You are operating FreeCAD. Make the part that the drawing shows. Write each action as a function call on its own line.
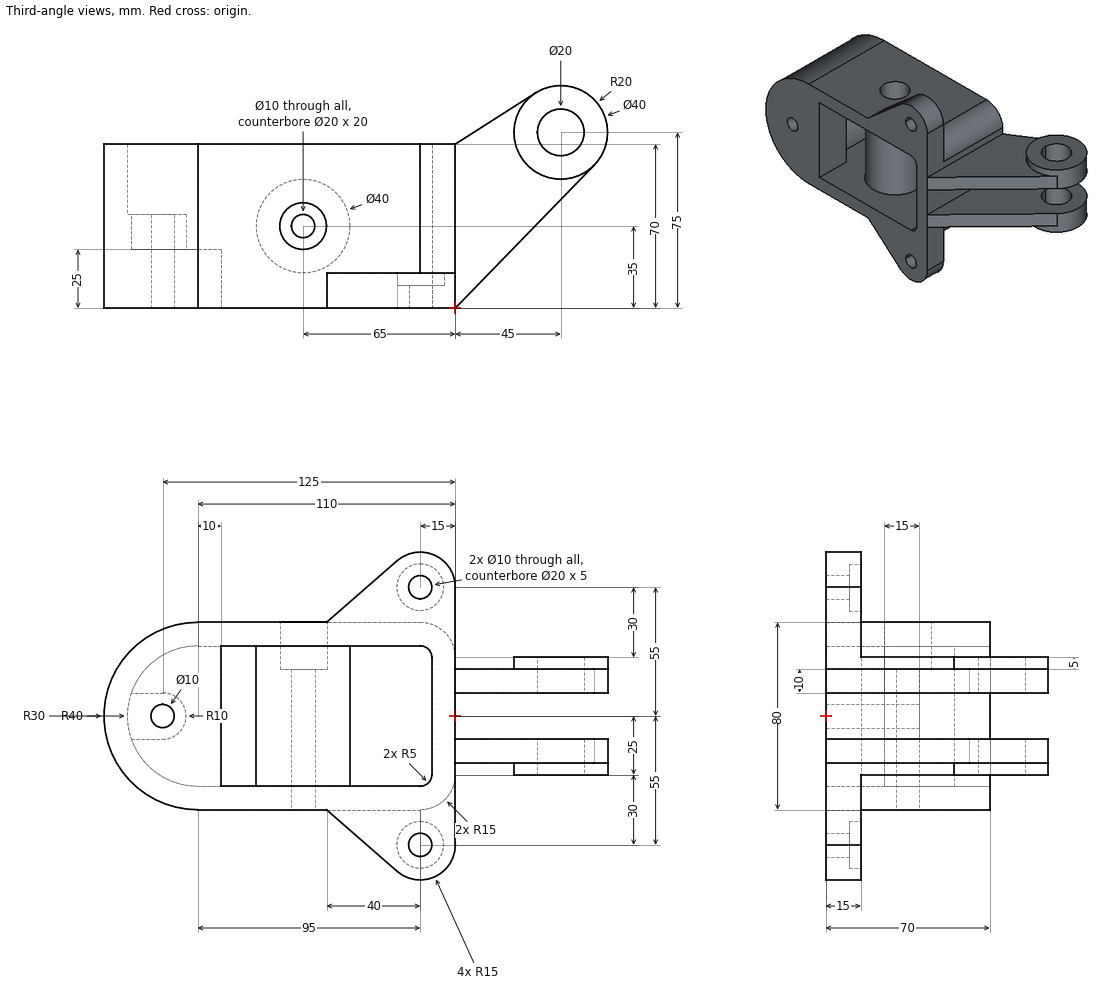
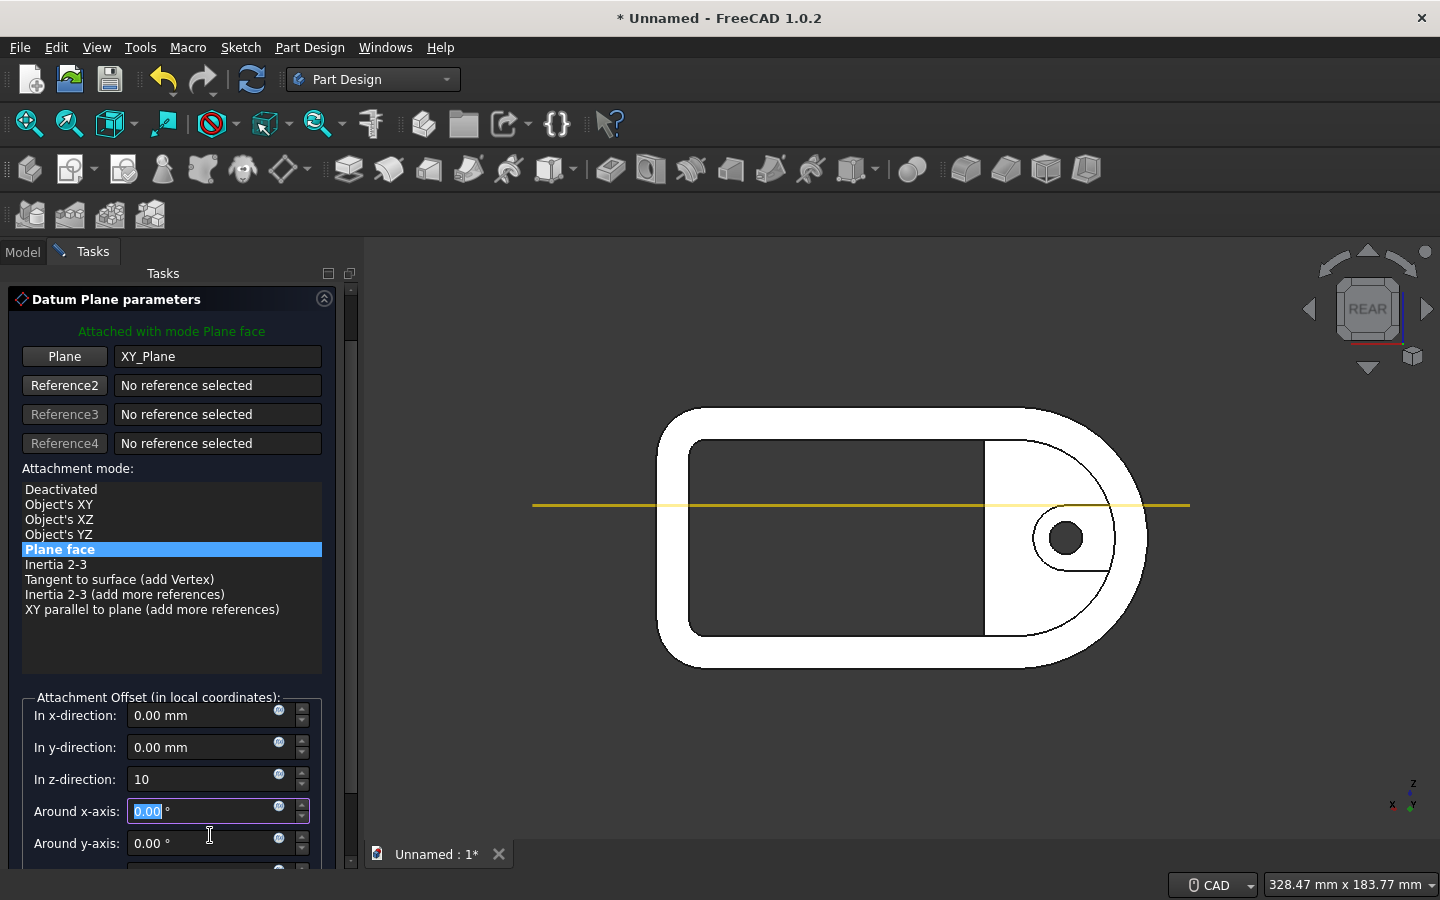
scroll(351, 576, up, 2)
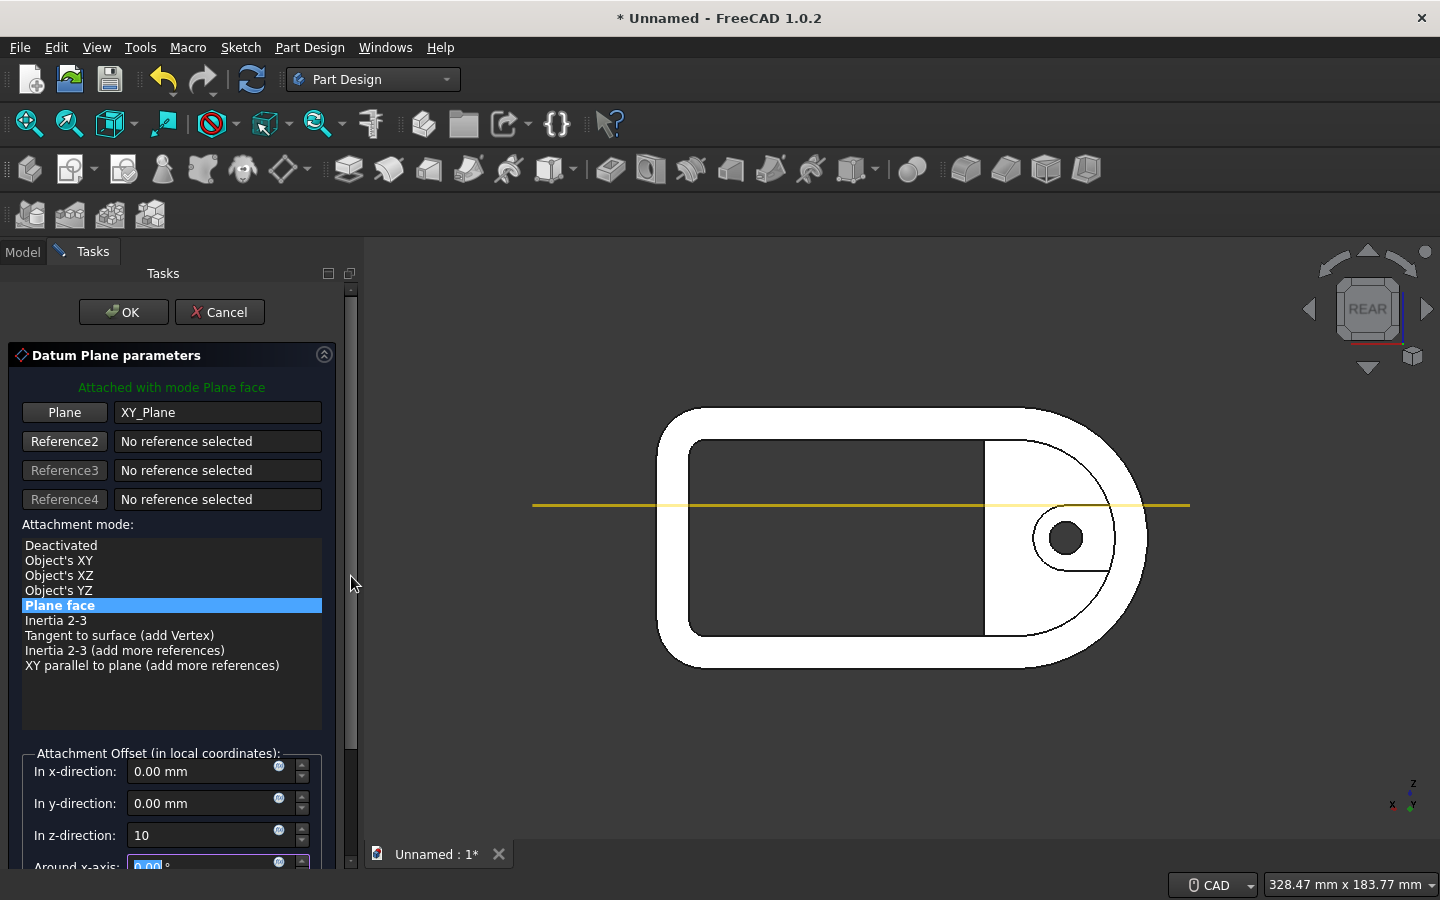
click(124, 312)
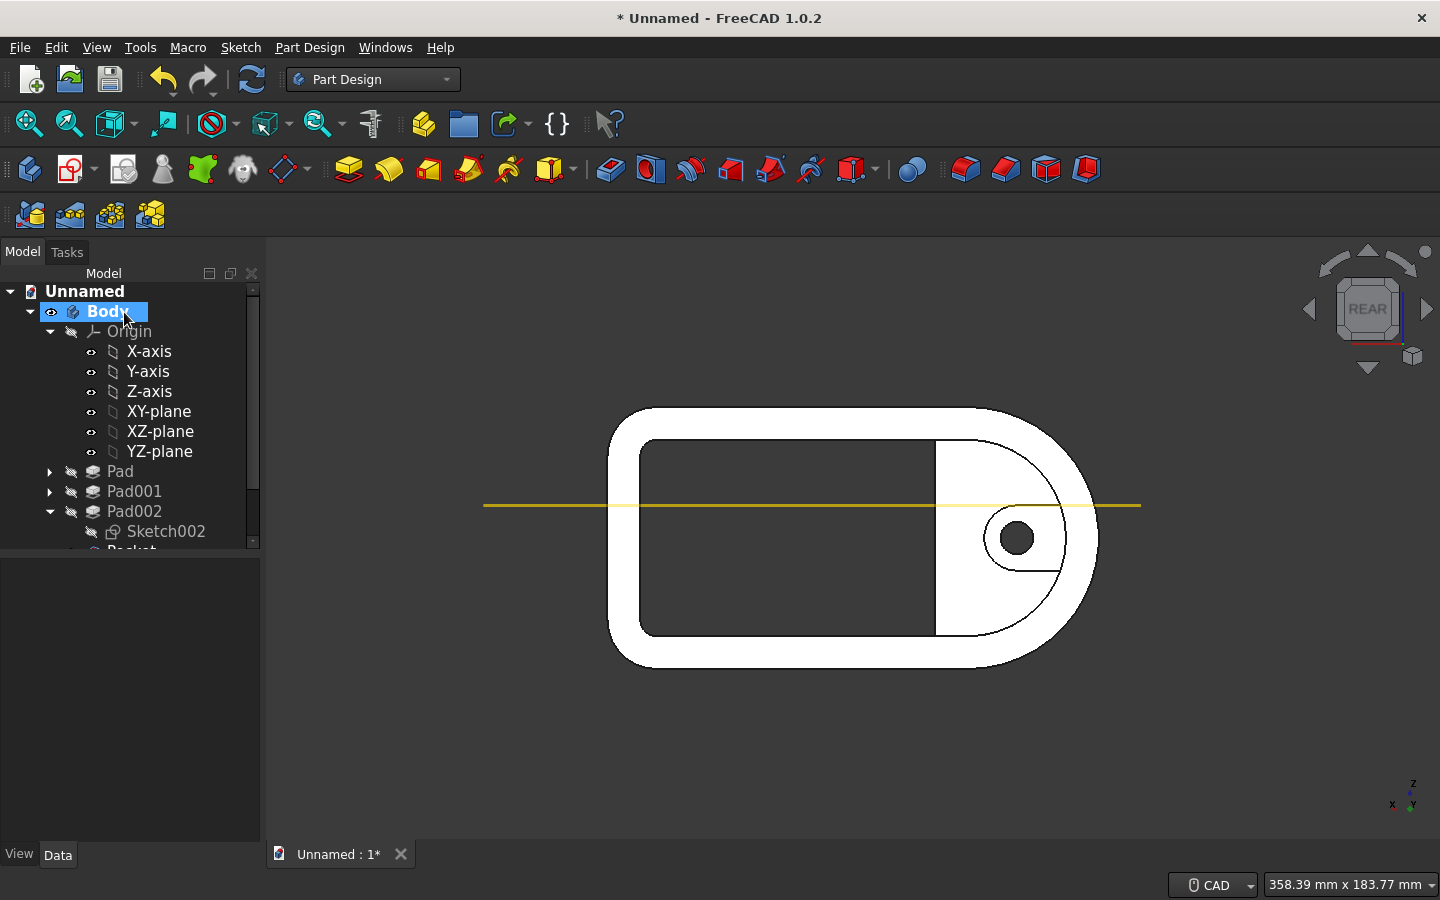
scroll(100, 407, down, 3)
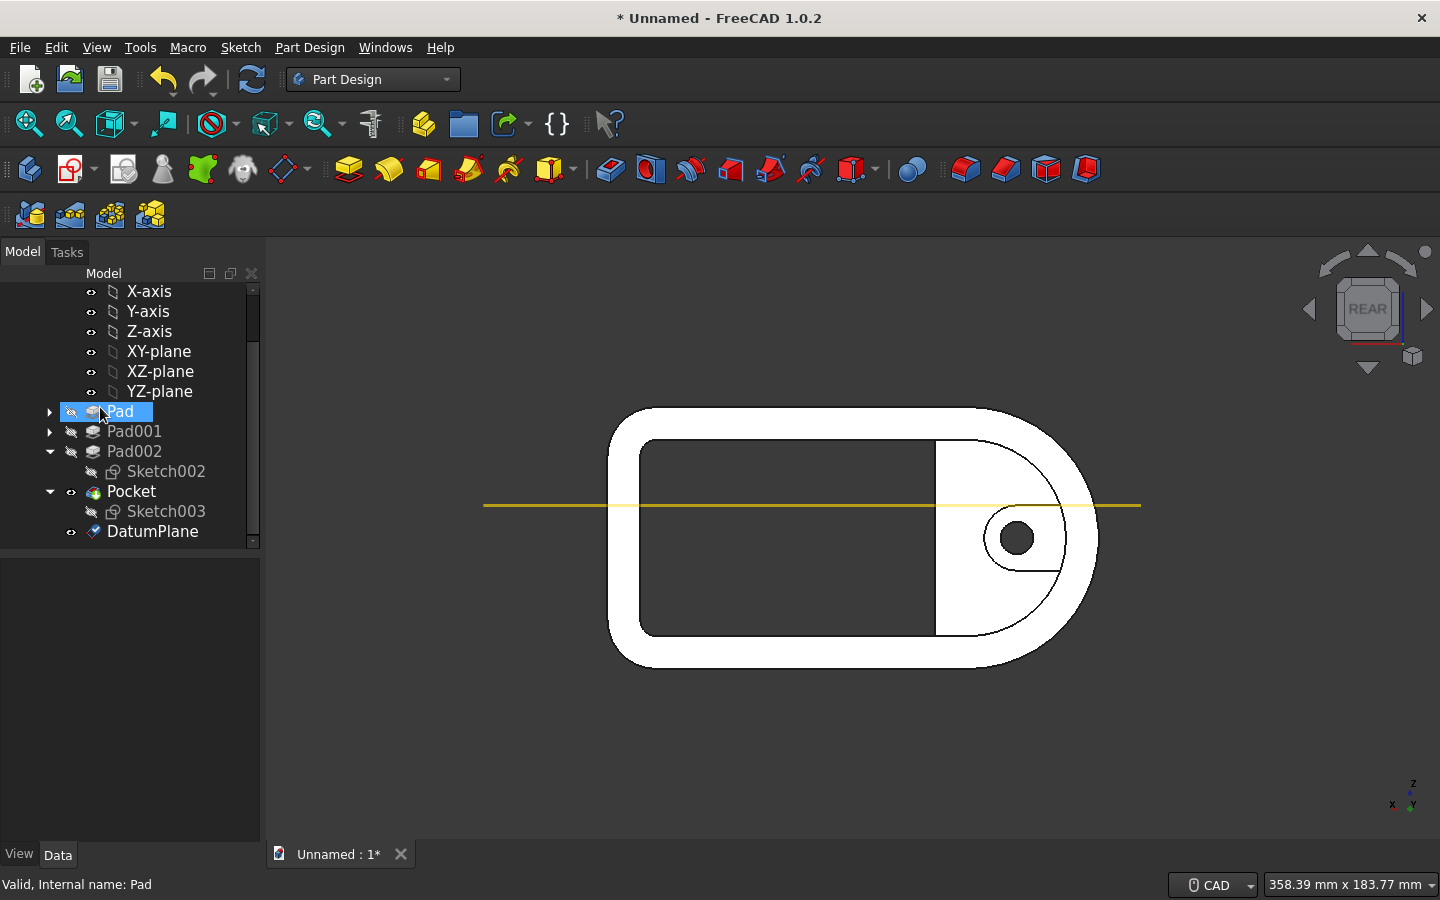
click(116, 532)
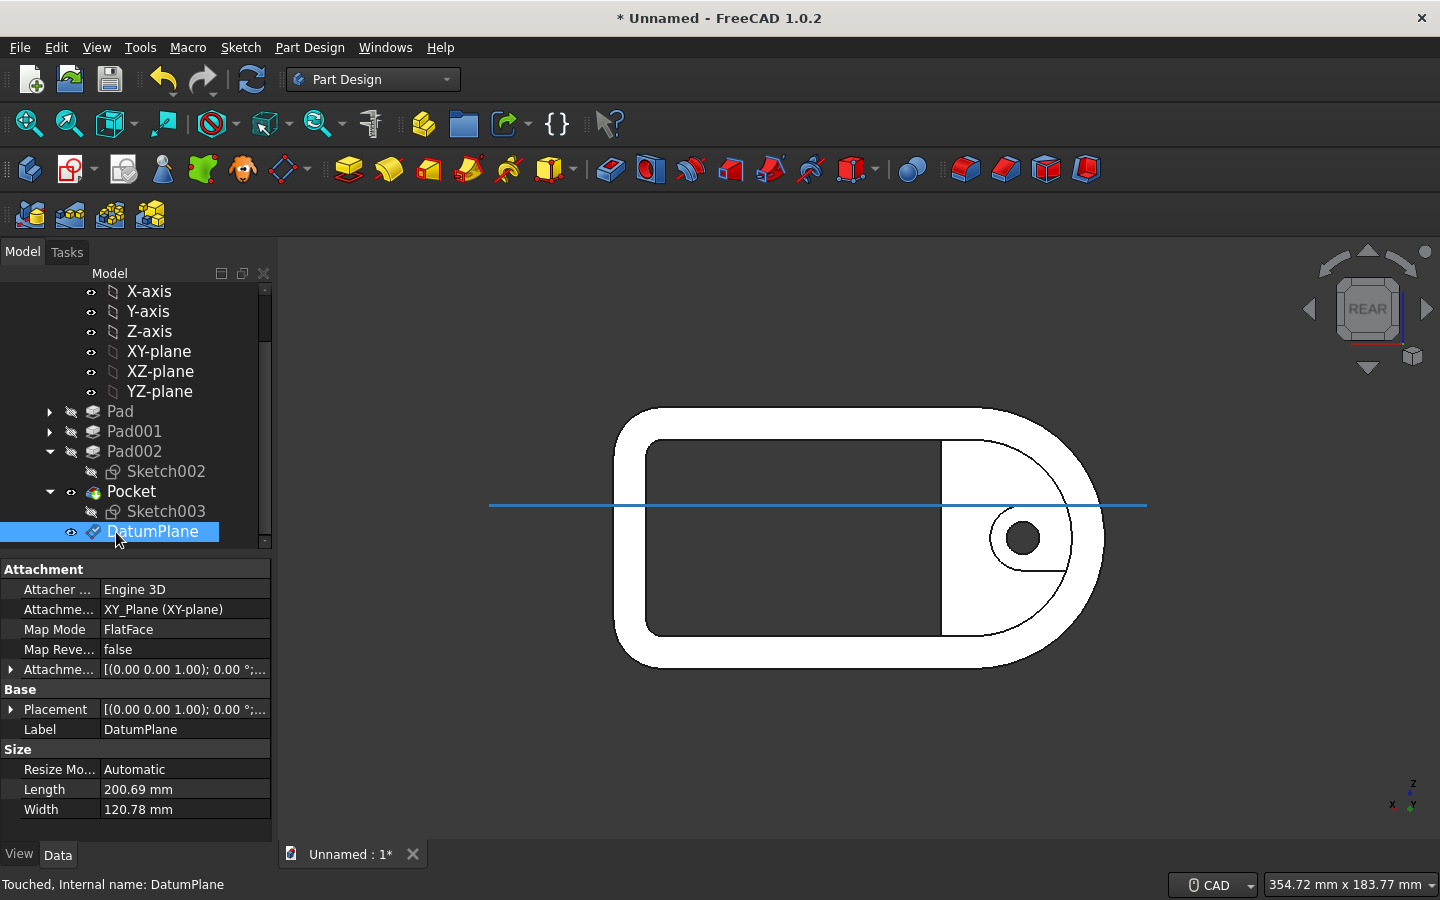
click(70, 170)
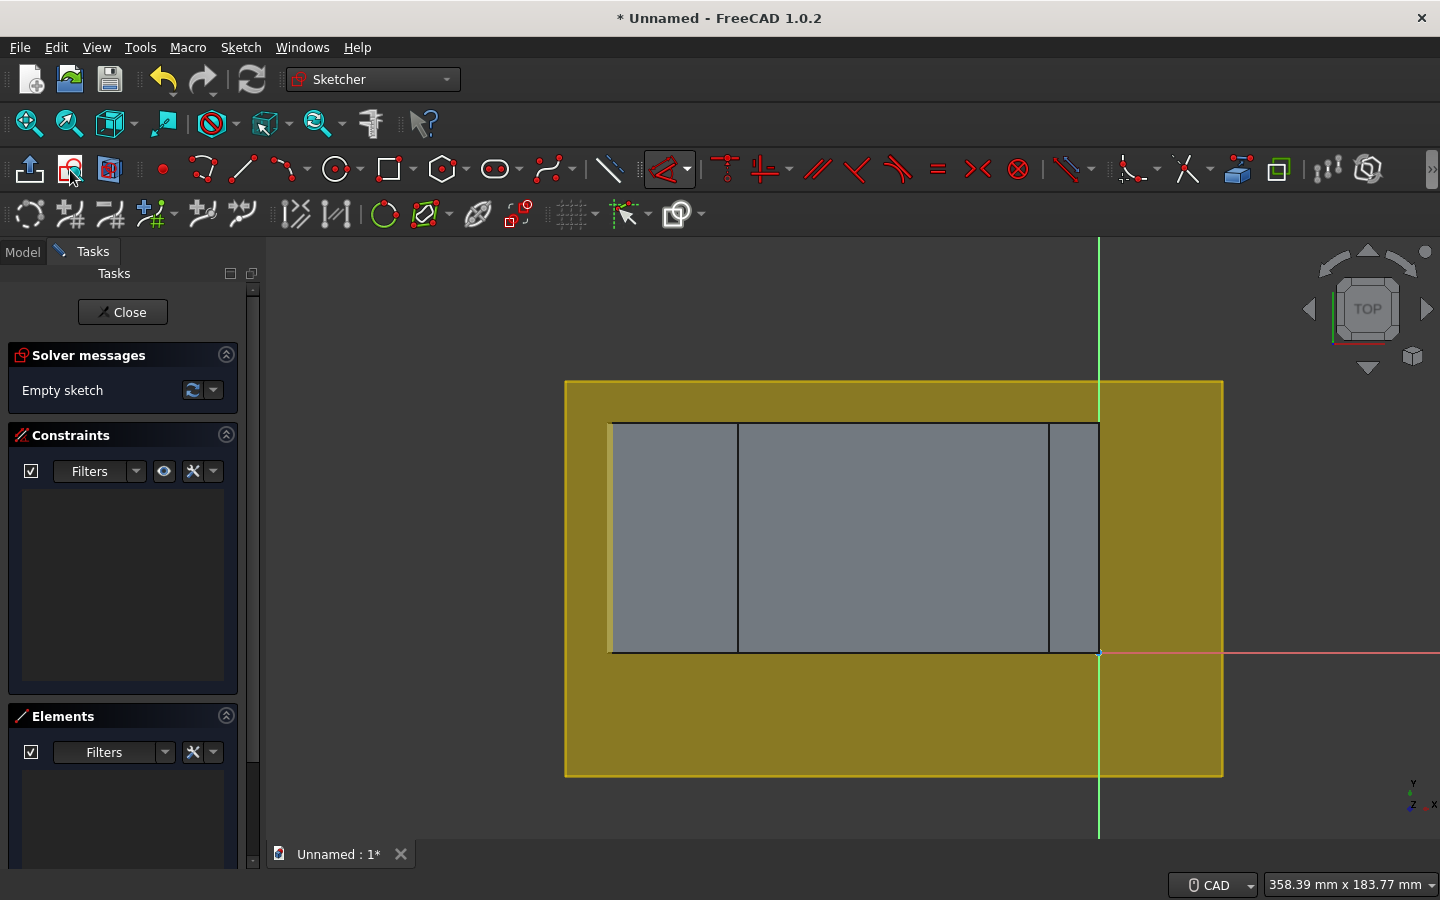
key(q)
key(s)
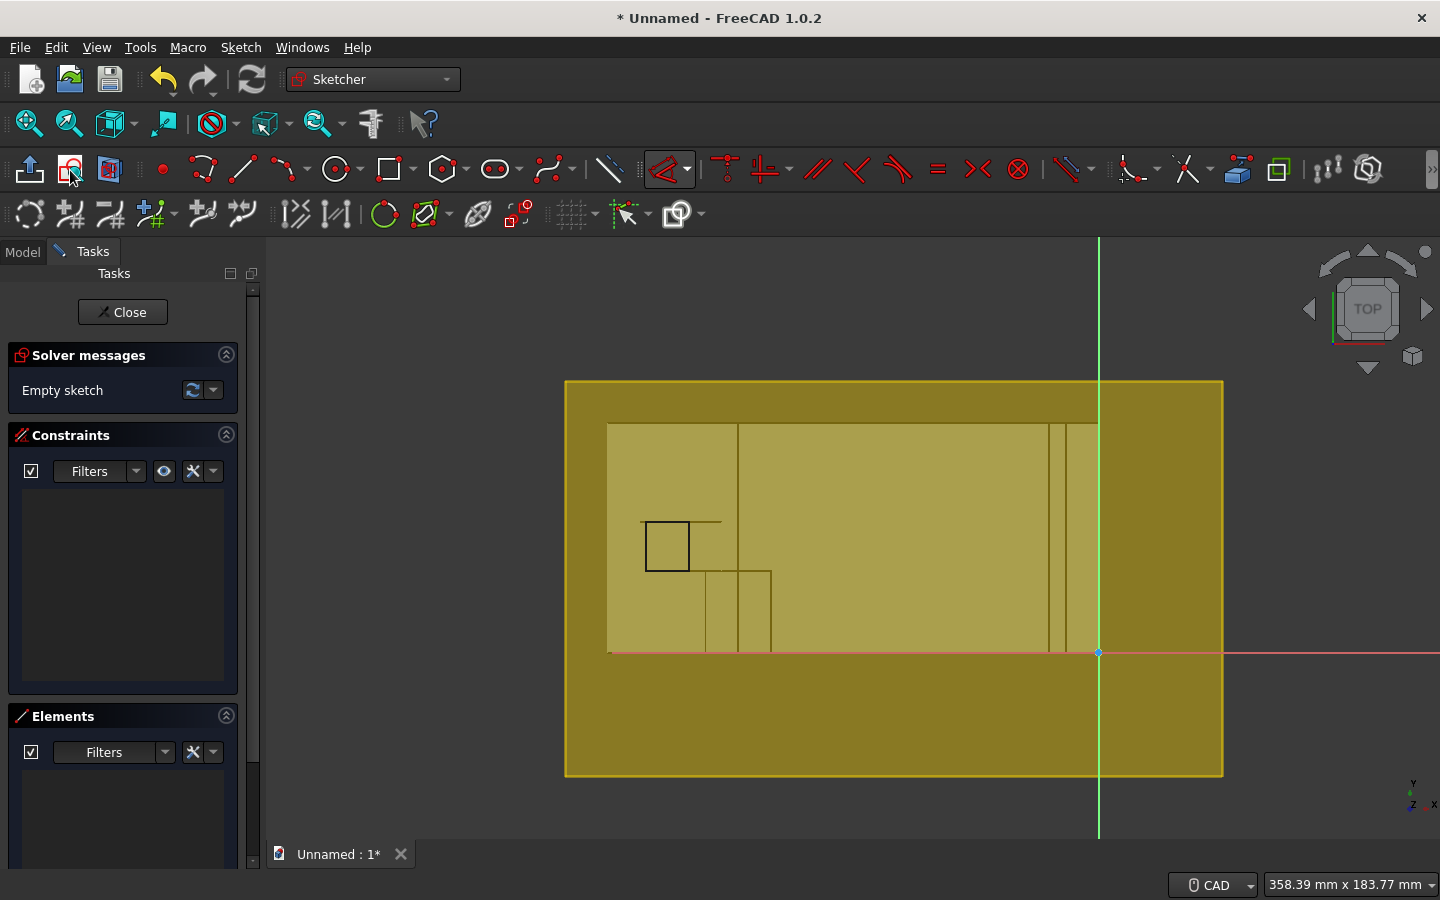
scroll(294, 700, down, 1)